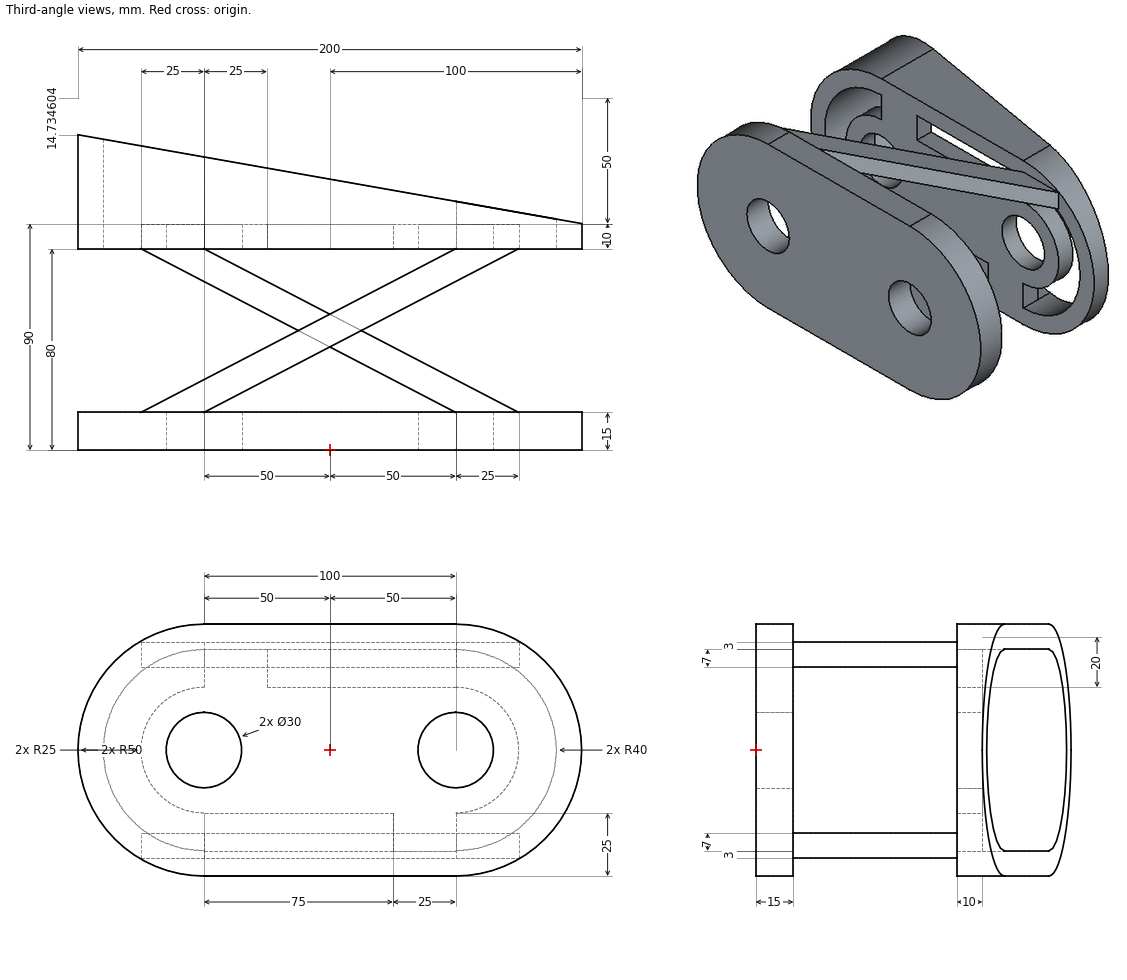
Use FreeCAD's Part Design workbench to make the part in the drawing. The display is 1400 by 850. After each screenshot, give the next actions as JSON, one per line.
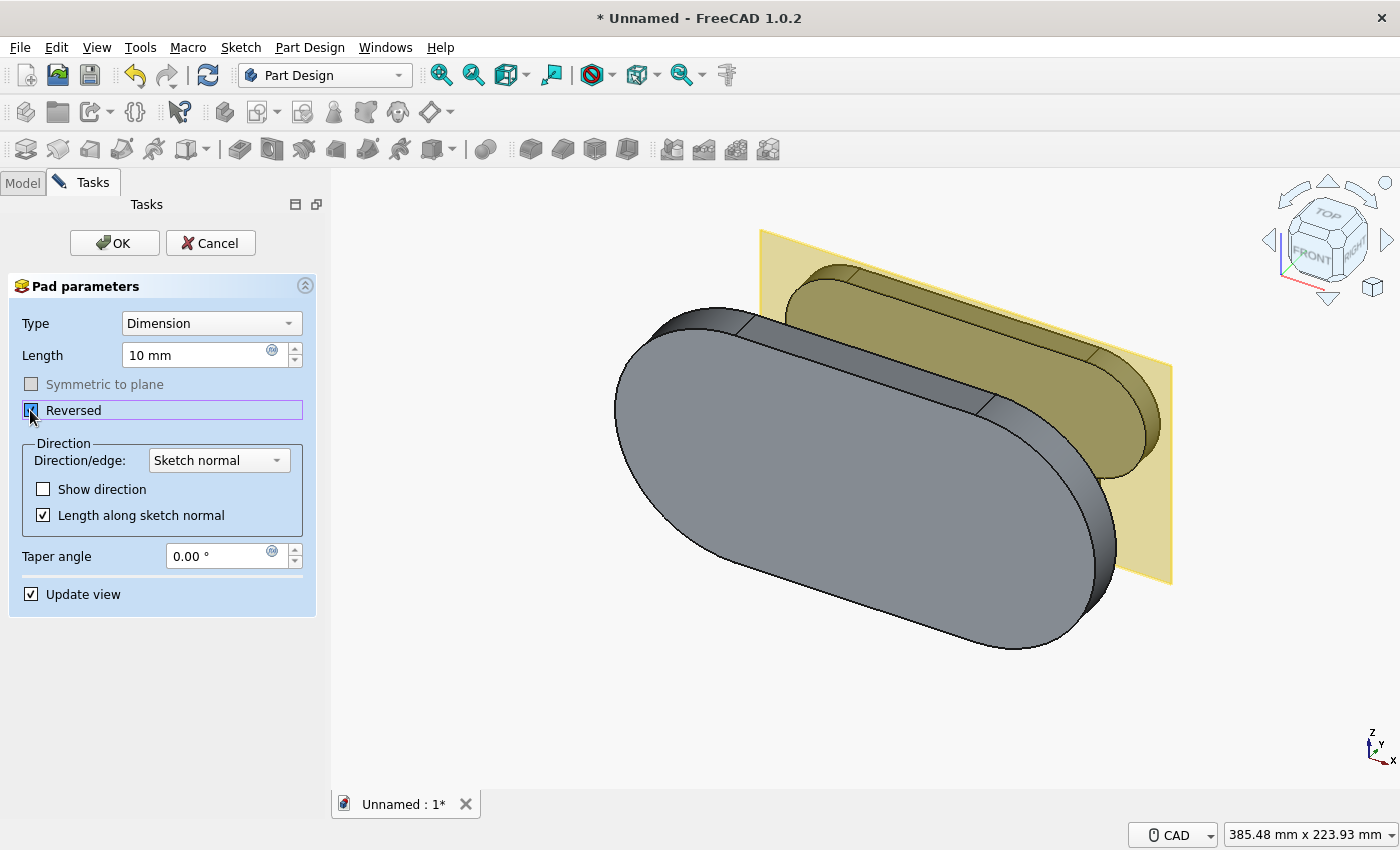
{"action": "left_click", "coordinate": [115, 243]}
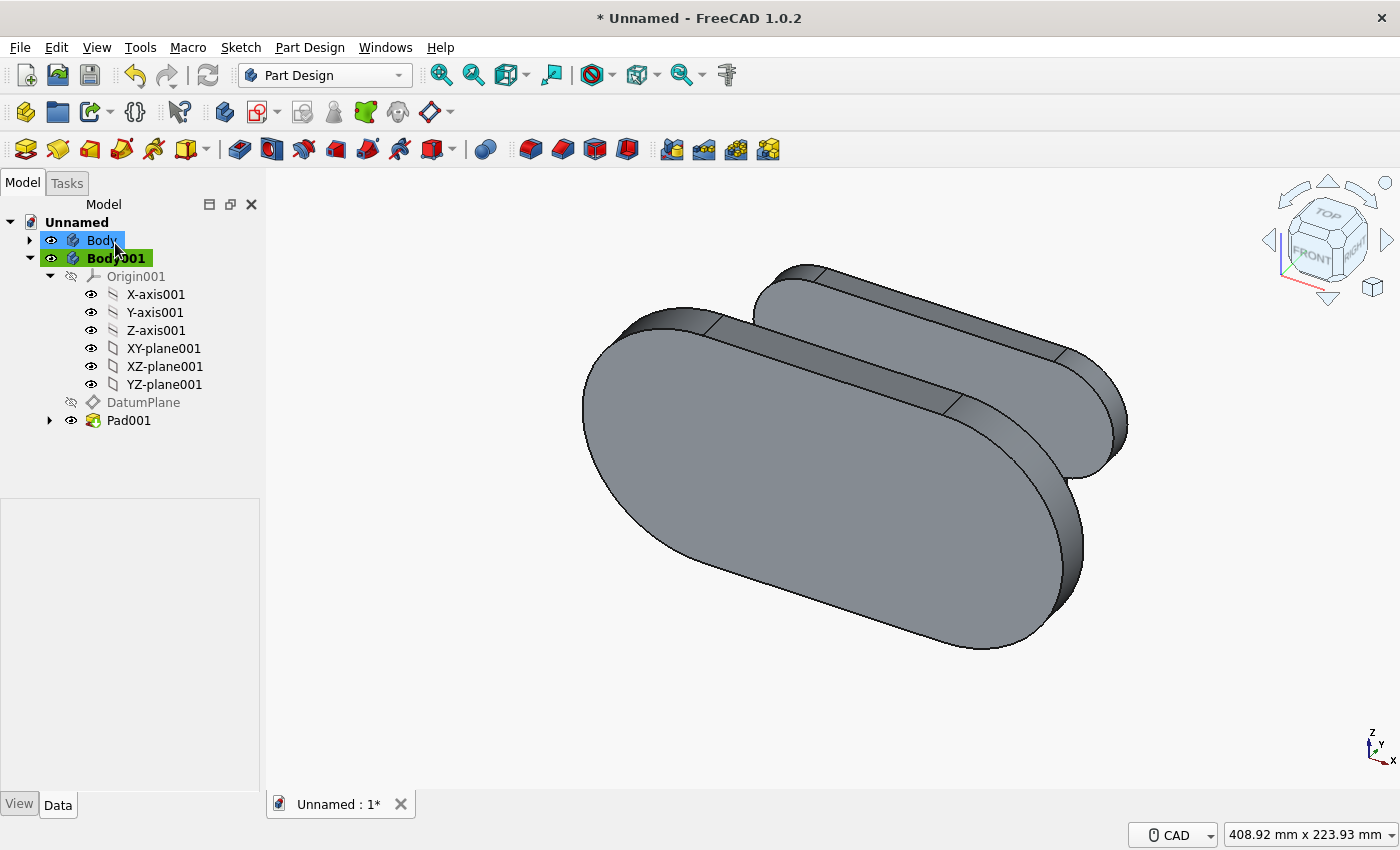
{"action": "key", "text": "4"}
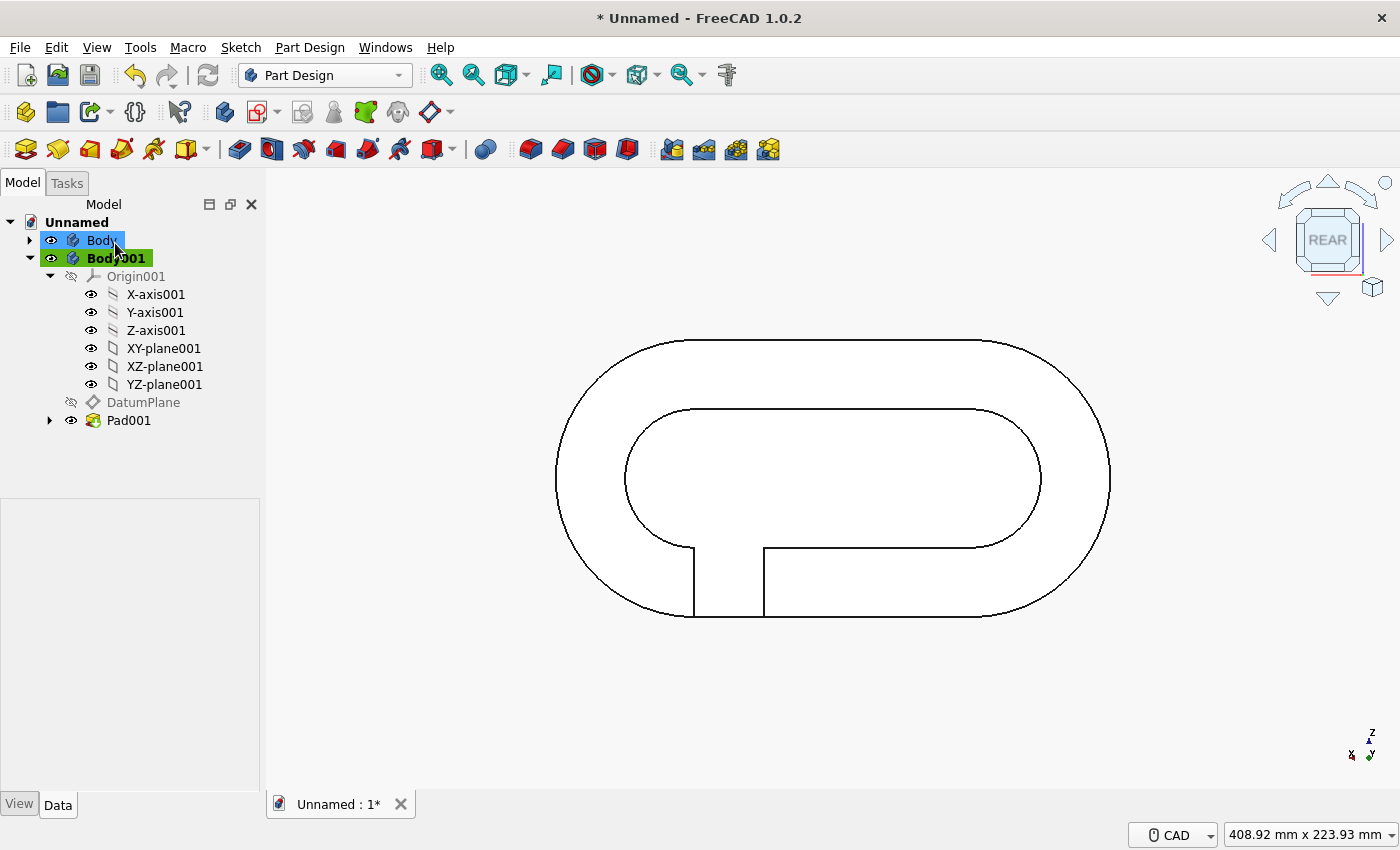
{"action": "left_click", "coordinate": [442, 76]}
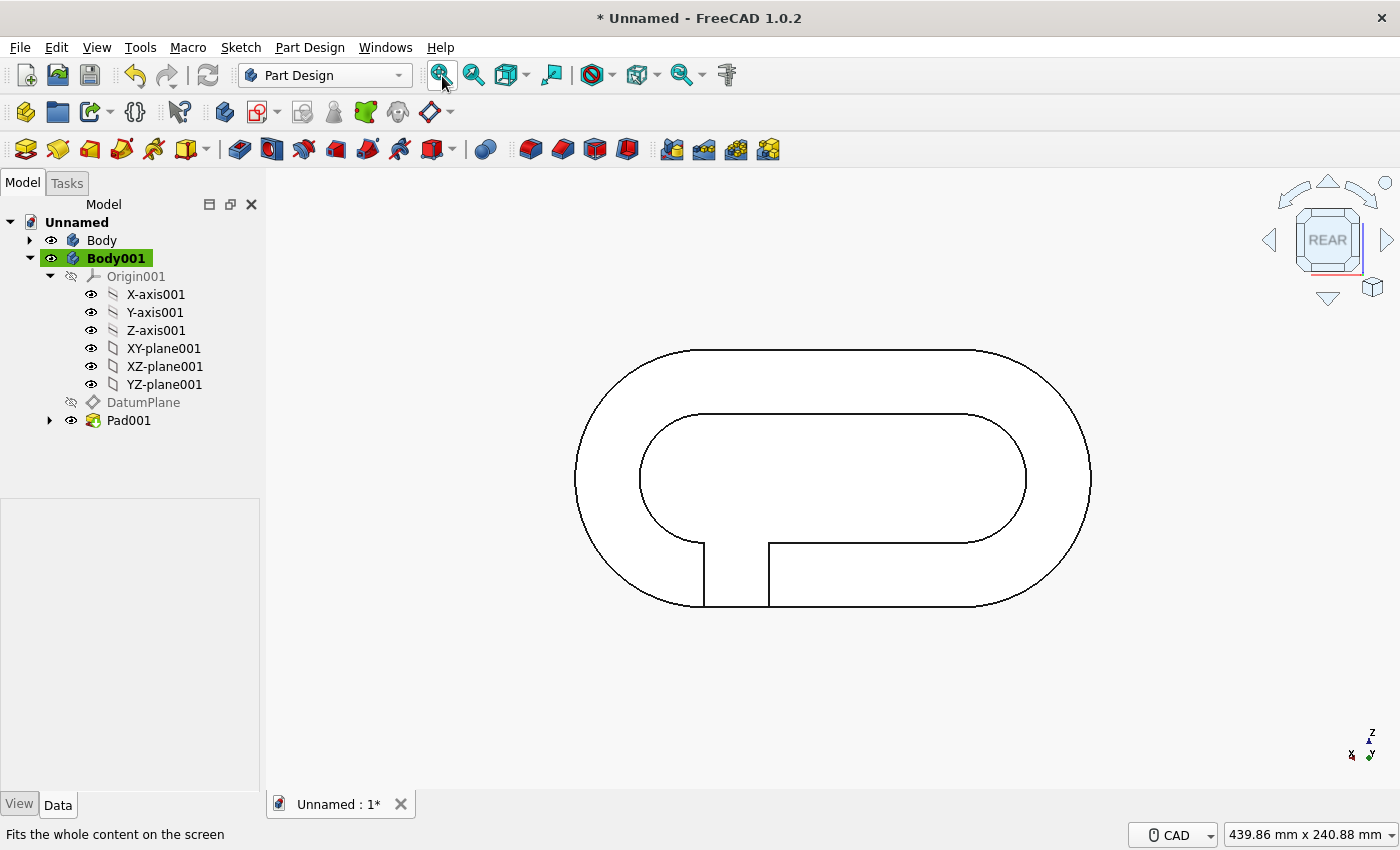
{"action": "left_click", "coordinate": [723, 482]}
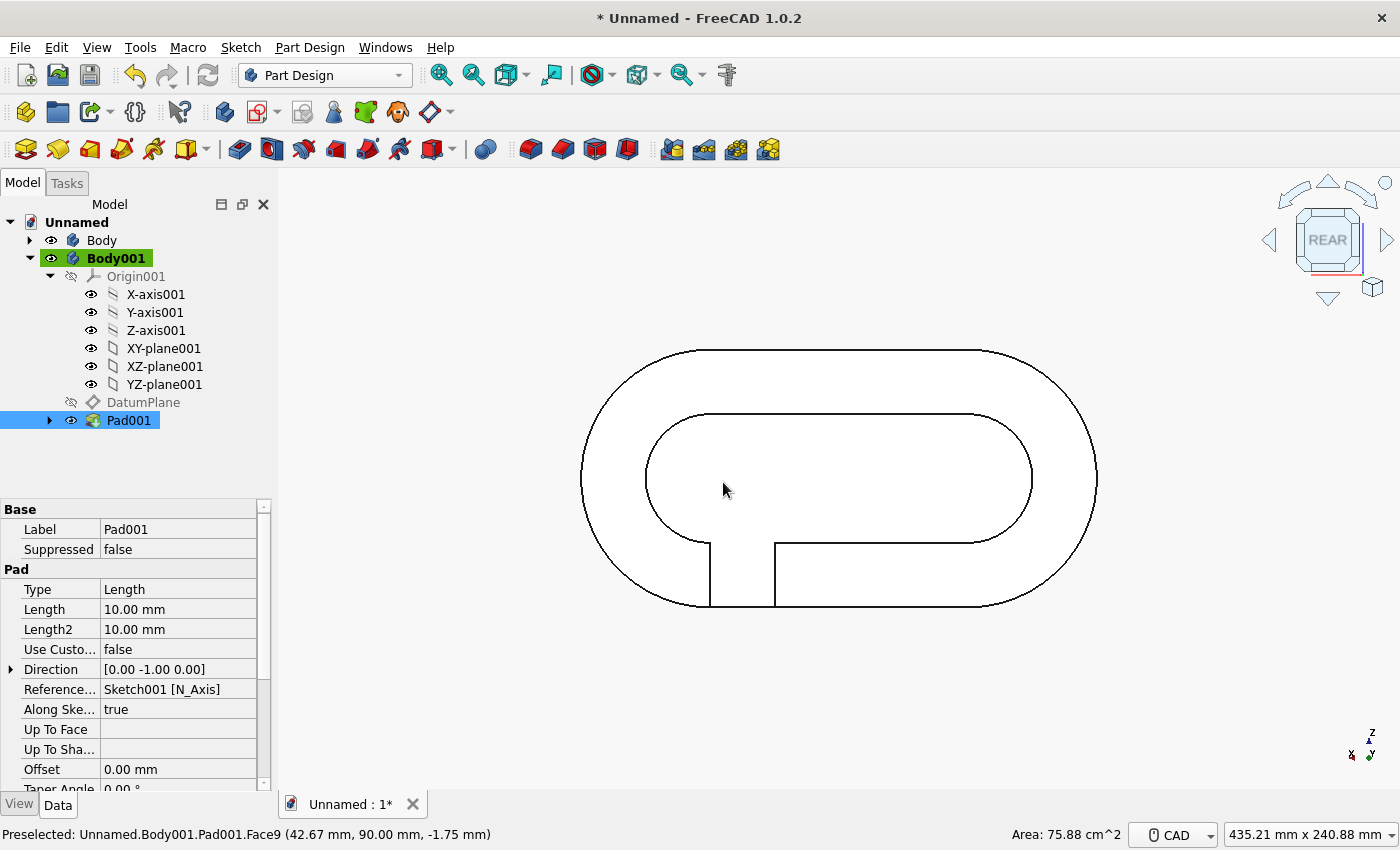
{"action": "left_click", "coordinate": [258, 112]}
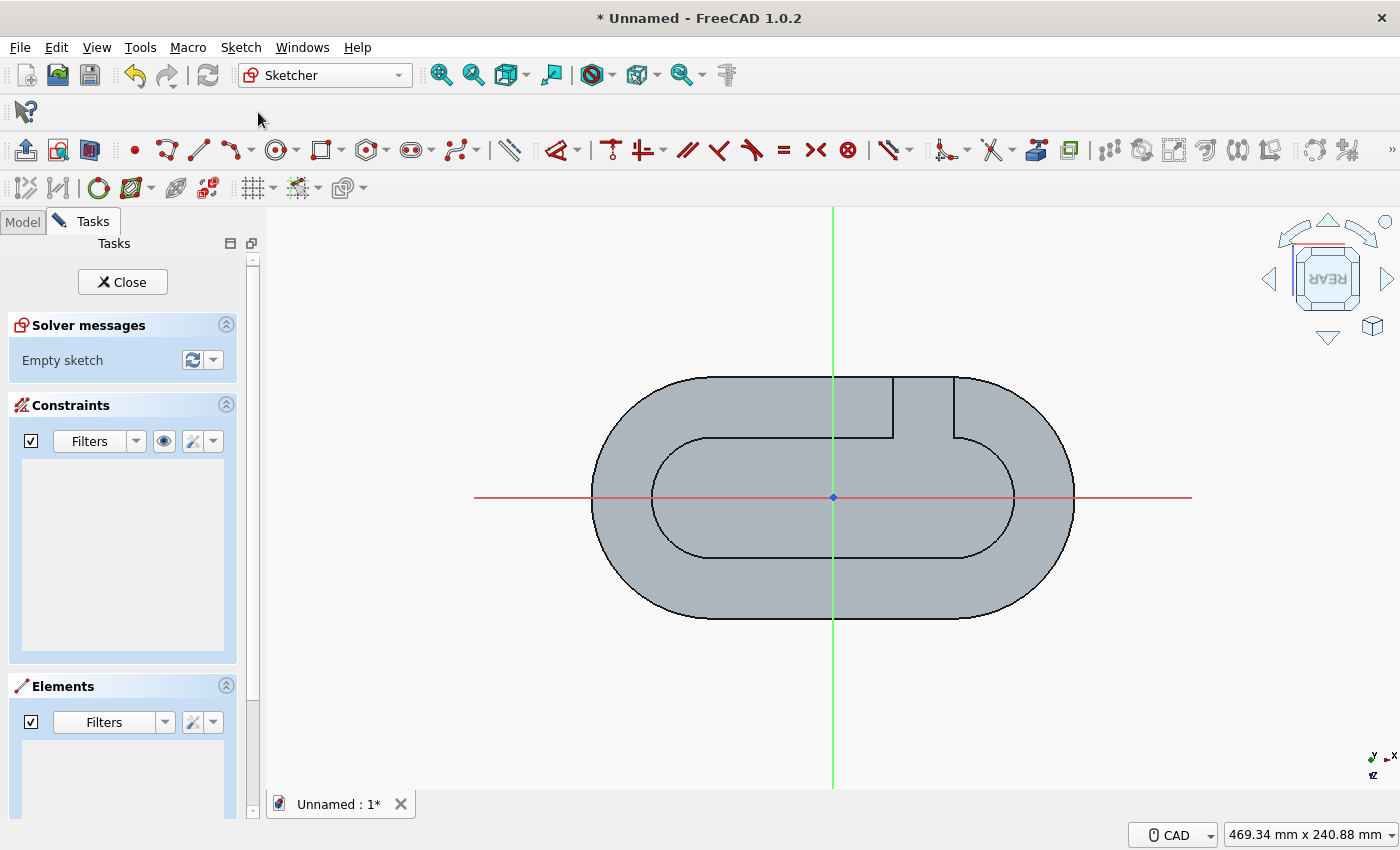
{"action": "scroll", "coordinate": [972, 498], "scroll_direction": "up", "scroll_amount": 2}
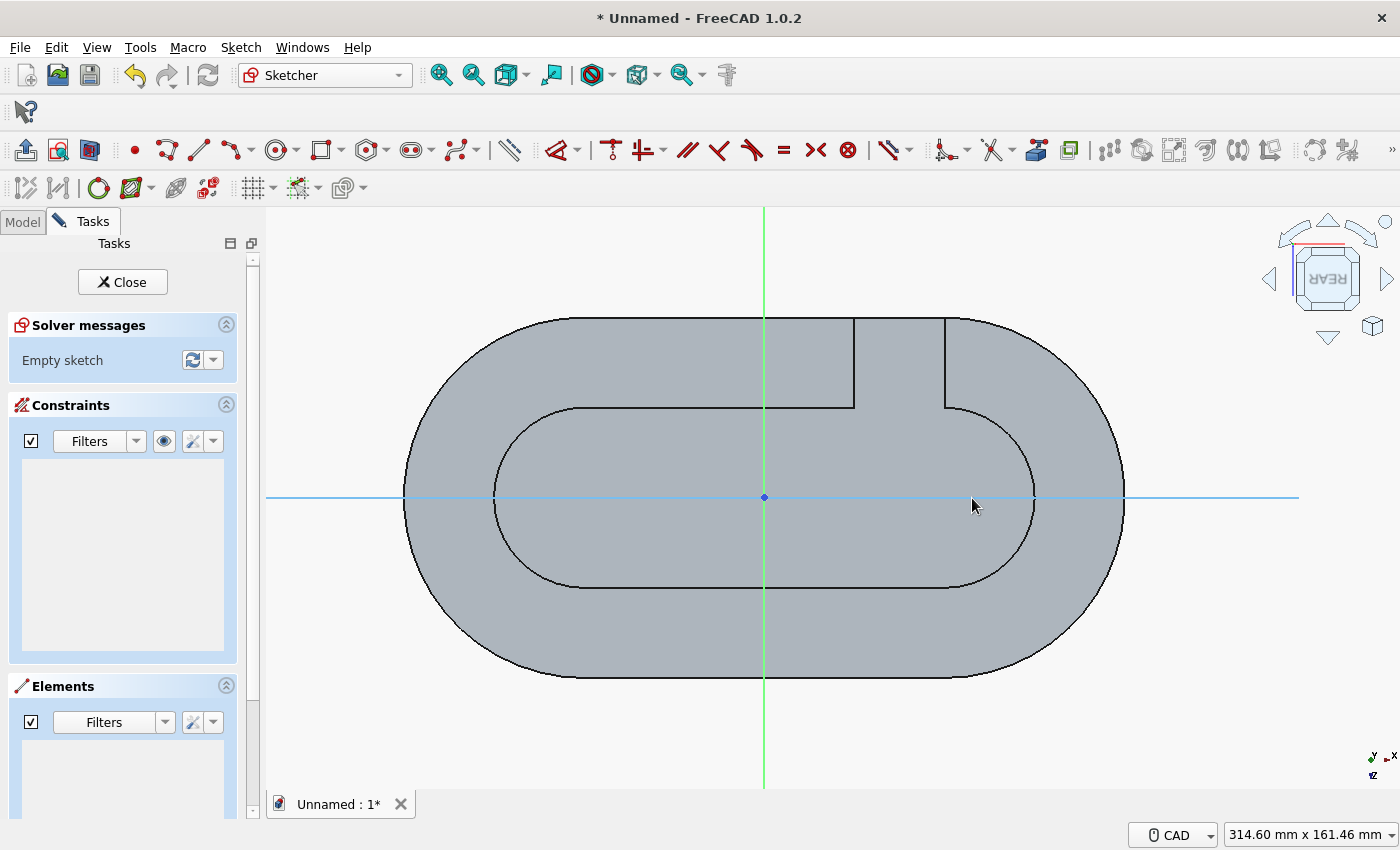
{"action": "left_click", "coordinate": [412, 150]}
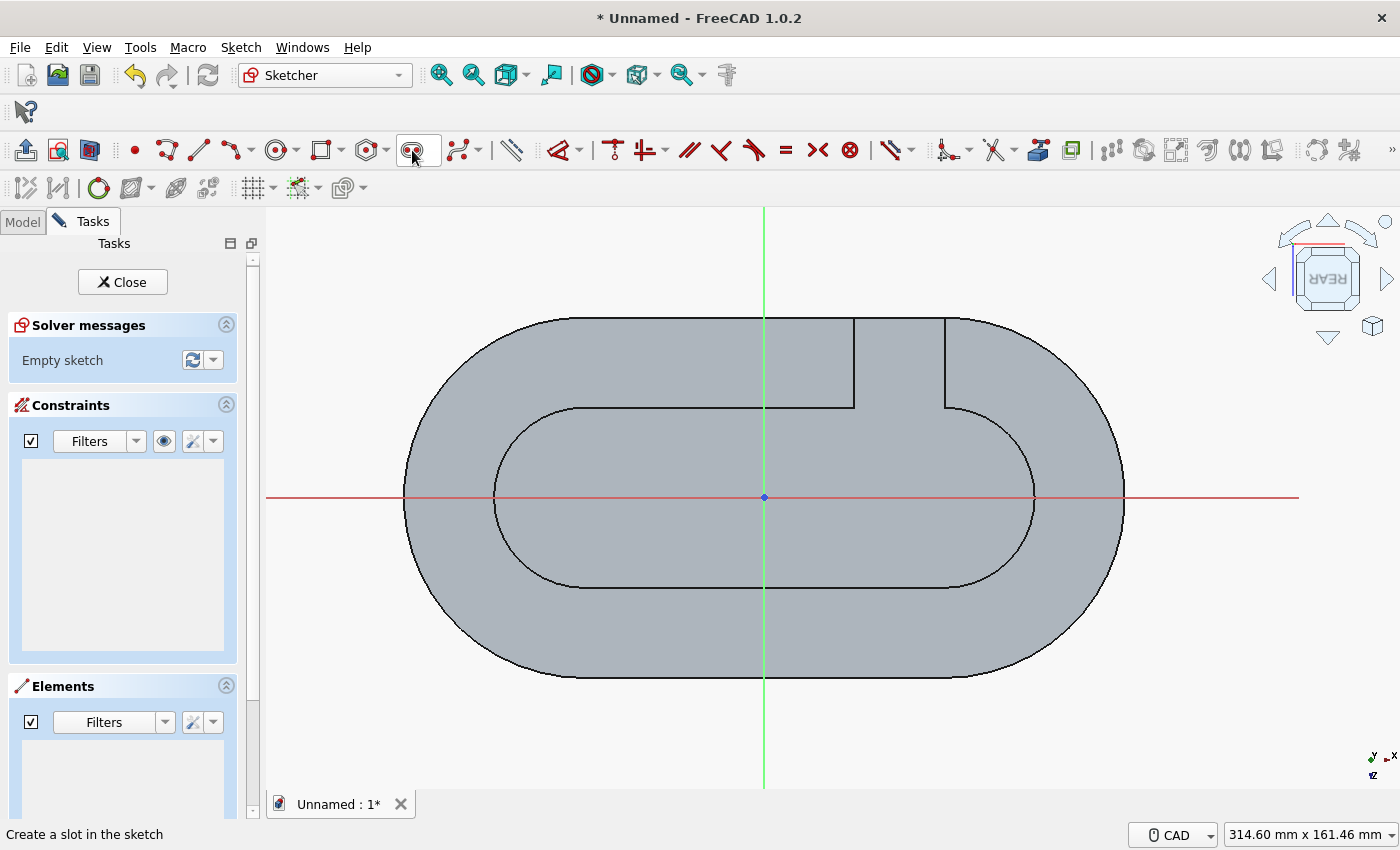
{"action": "left_click", "coordinate": [584, 498]}